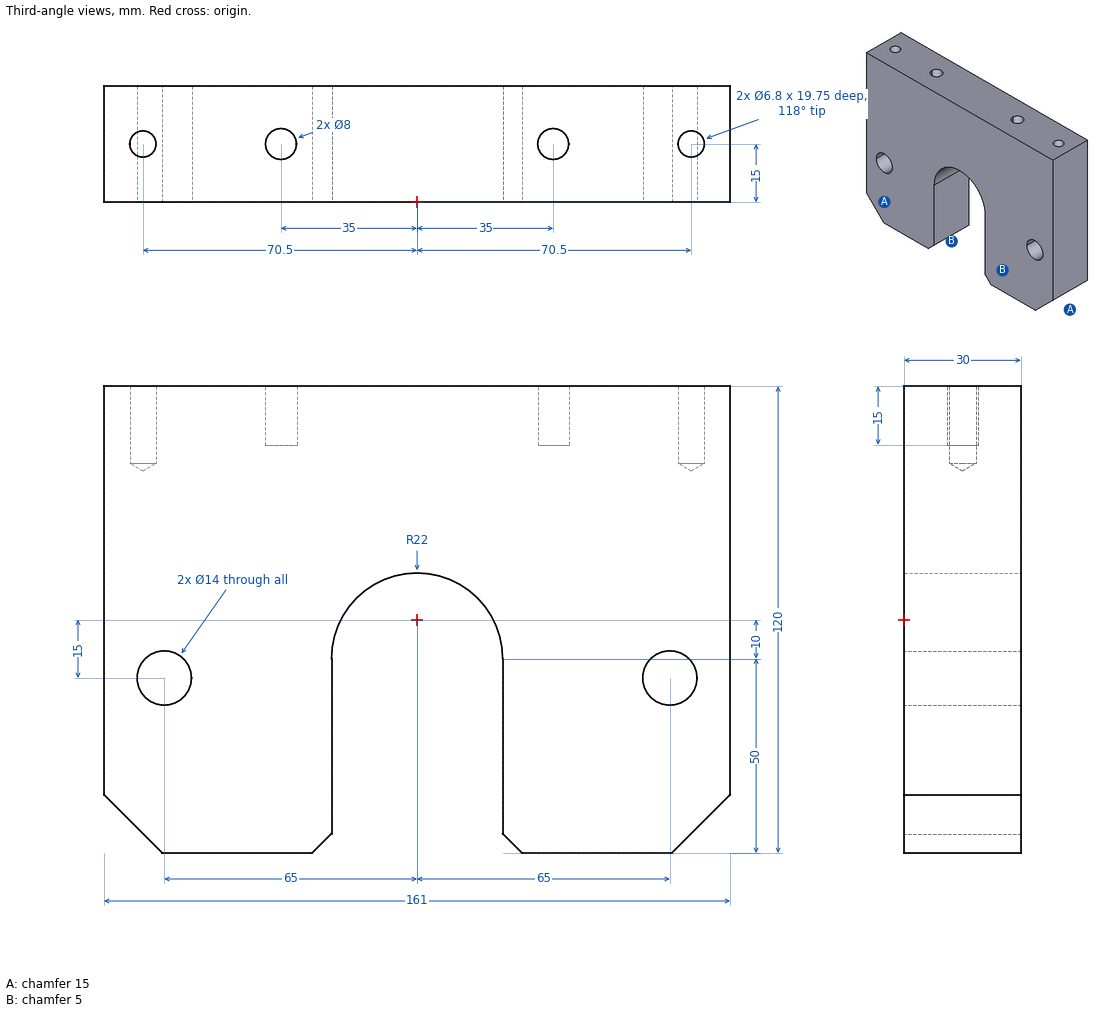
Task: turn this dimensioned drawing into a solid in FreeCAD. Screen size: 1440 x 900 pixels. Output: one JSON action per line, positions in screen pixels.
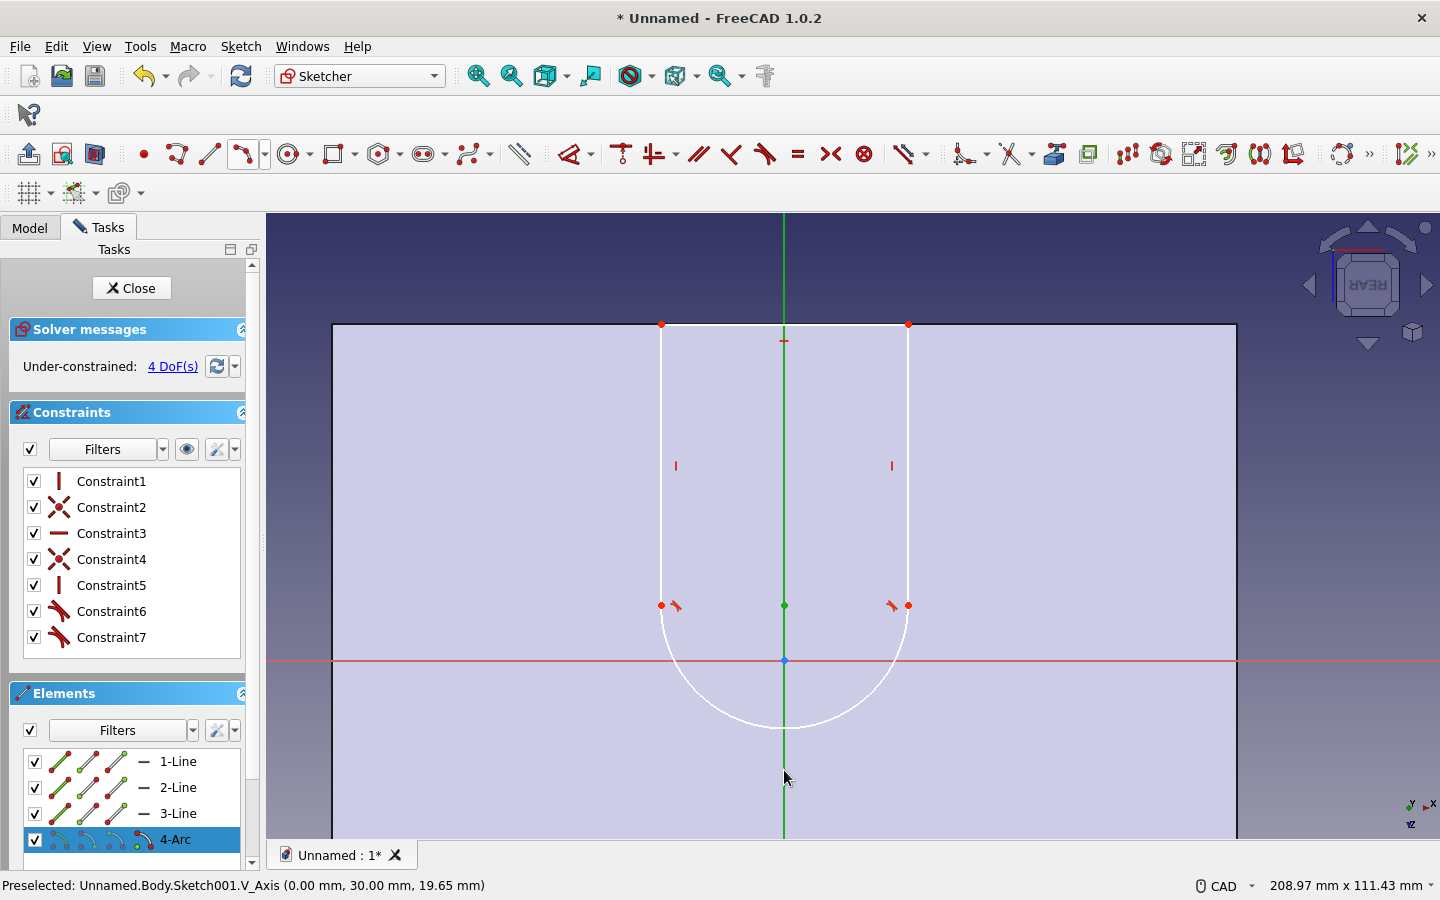
{"action": "key", "text": "c"}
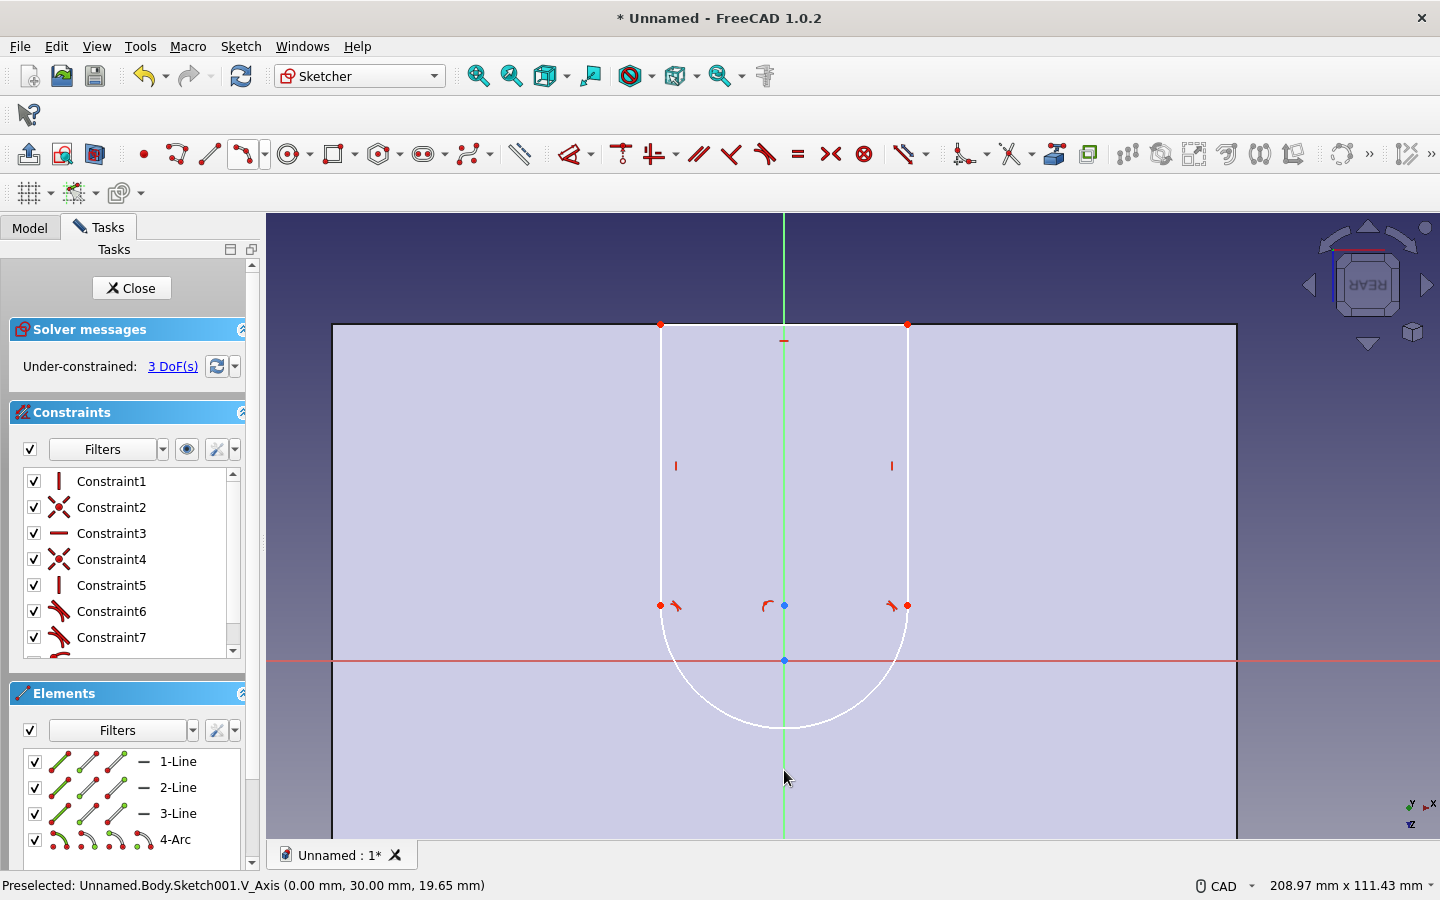
{"action": "key", "text": "d"}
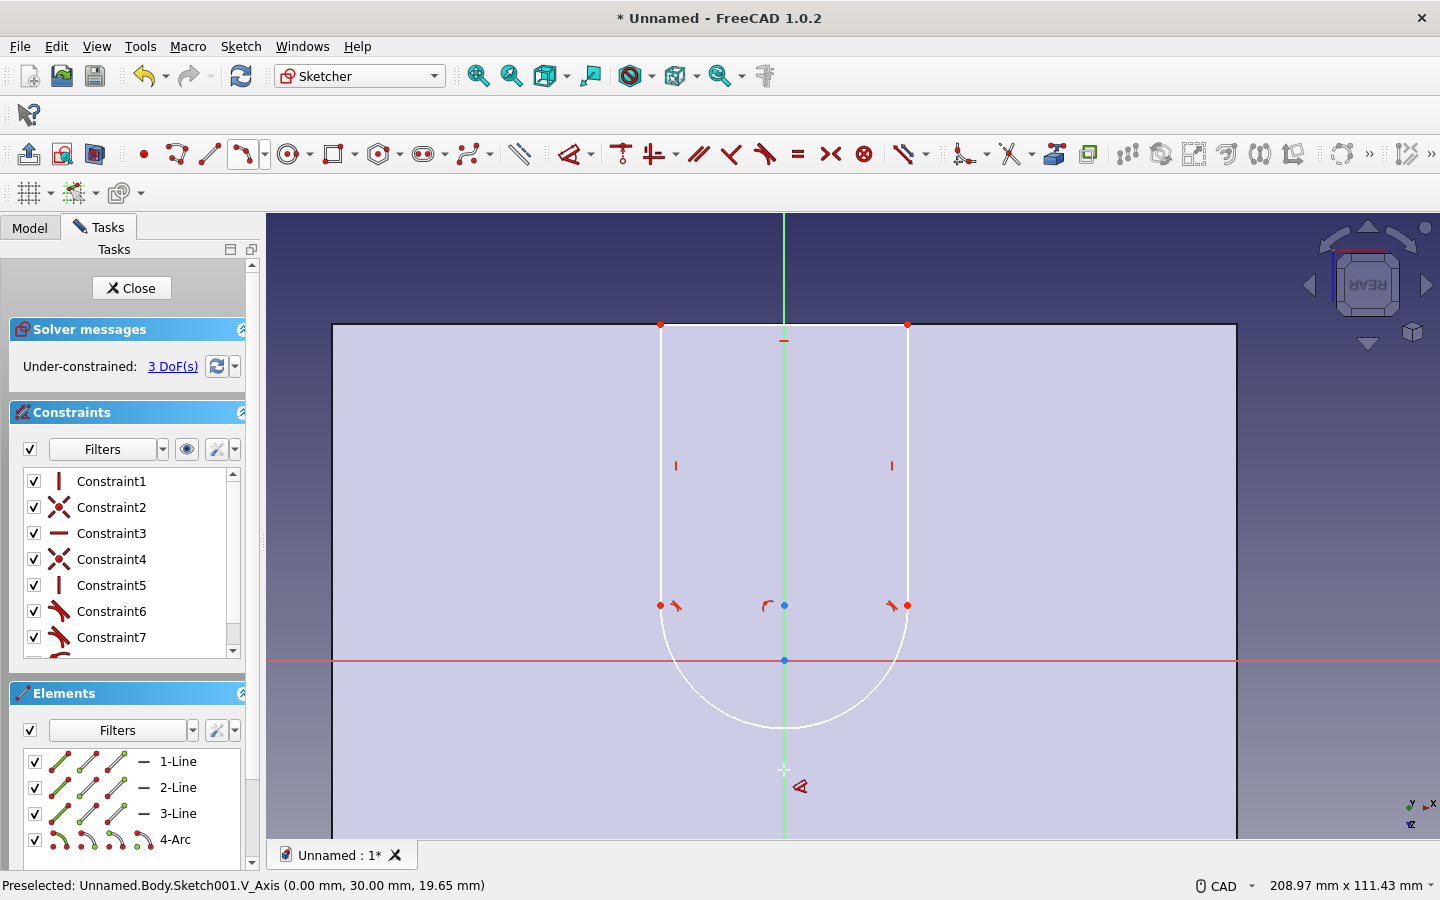
{"action": "left_click", "coordinate": [712, 705]}
{"action": "left_click", "coordinate": [693, 731]}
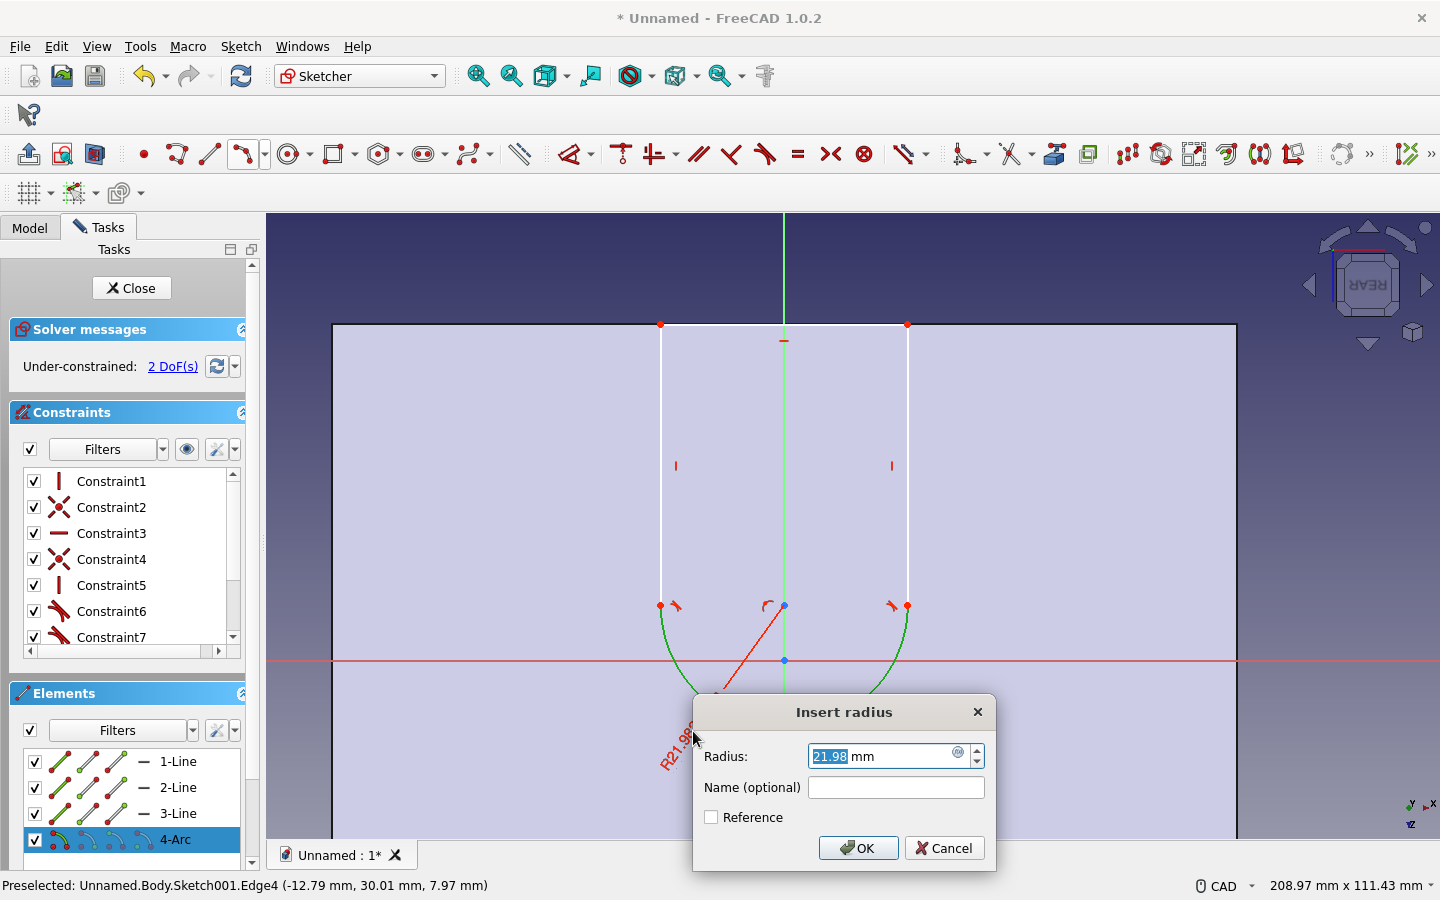
{"action": "type", "text": "22"}
{"action": "key", "text": "Return"}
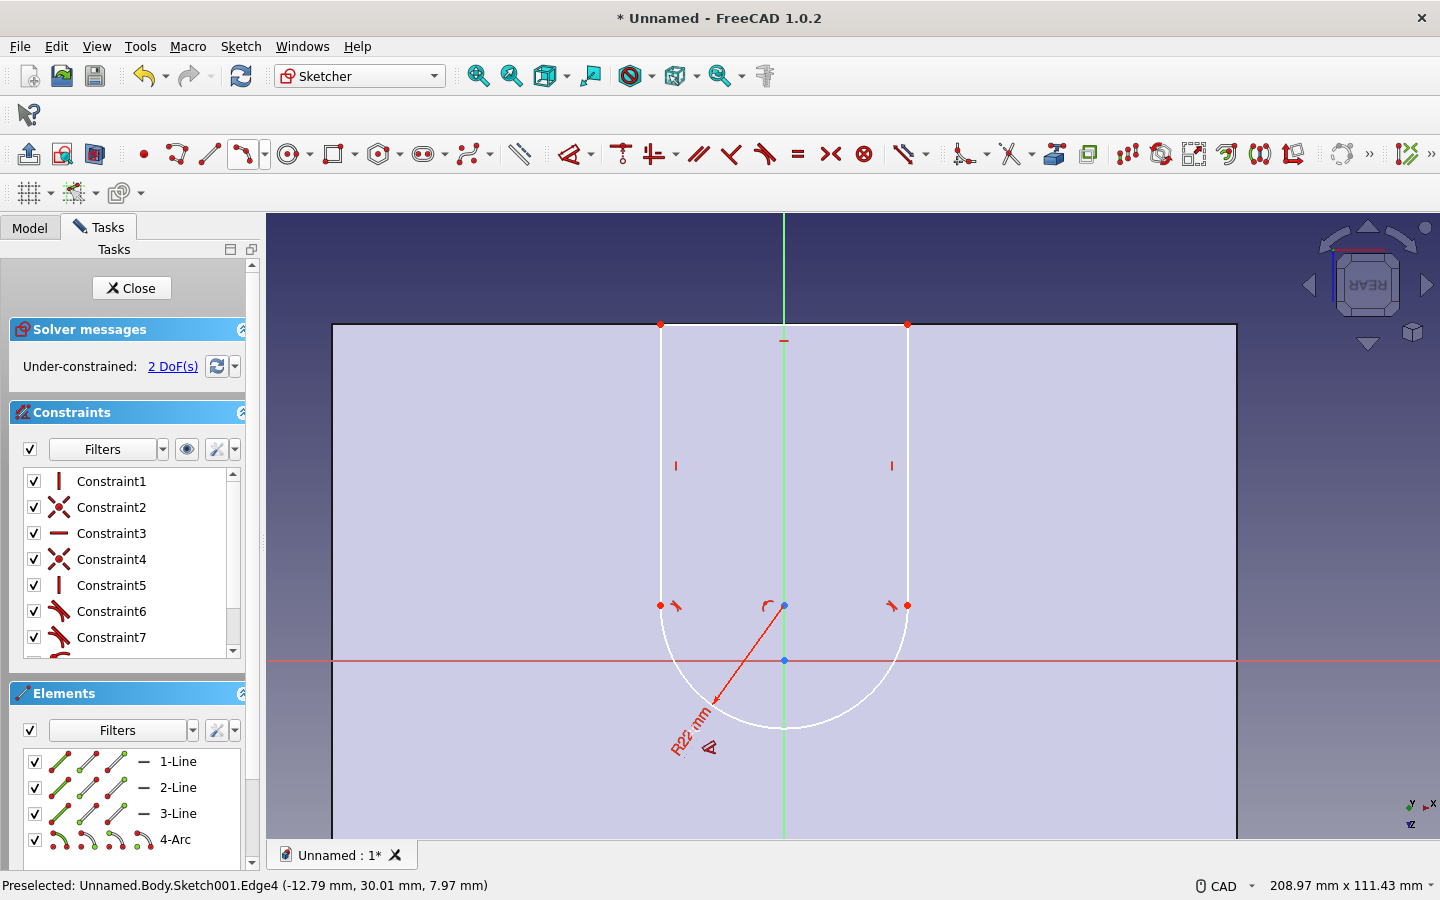
{"action": "left_click", "coordinate": [908, 521]}
{"action": "left_click", "coordinate": [942, 465]}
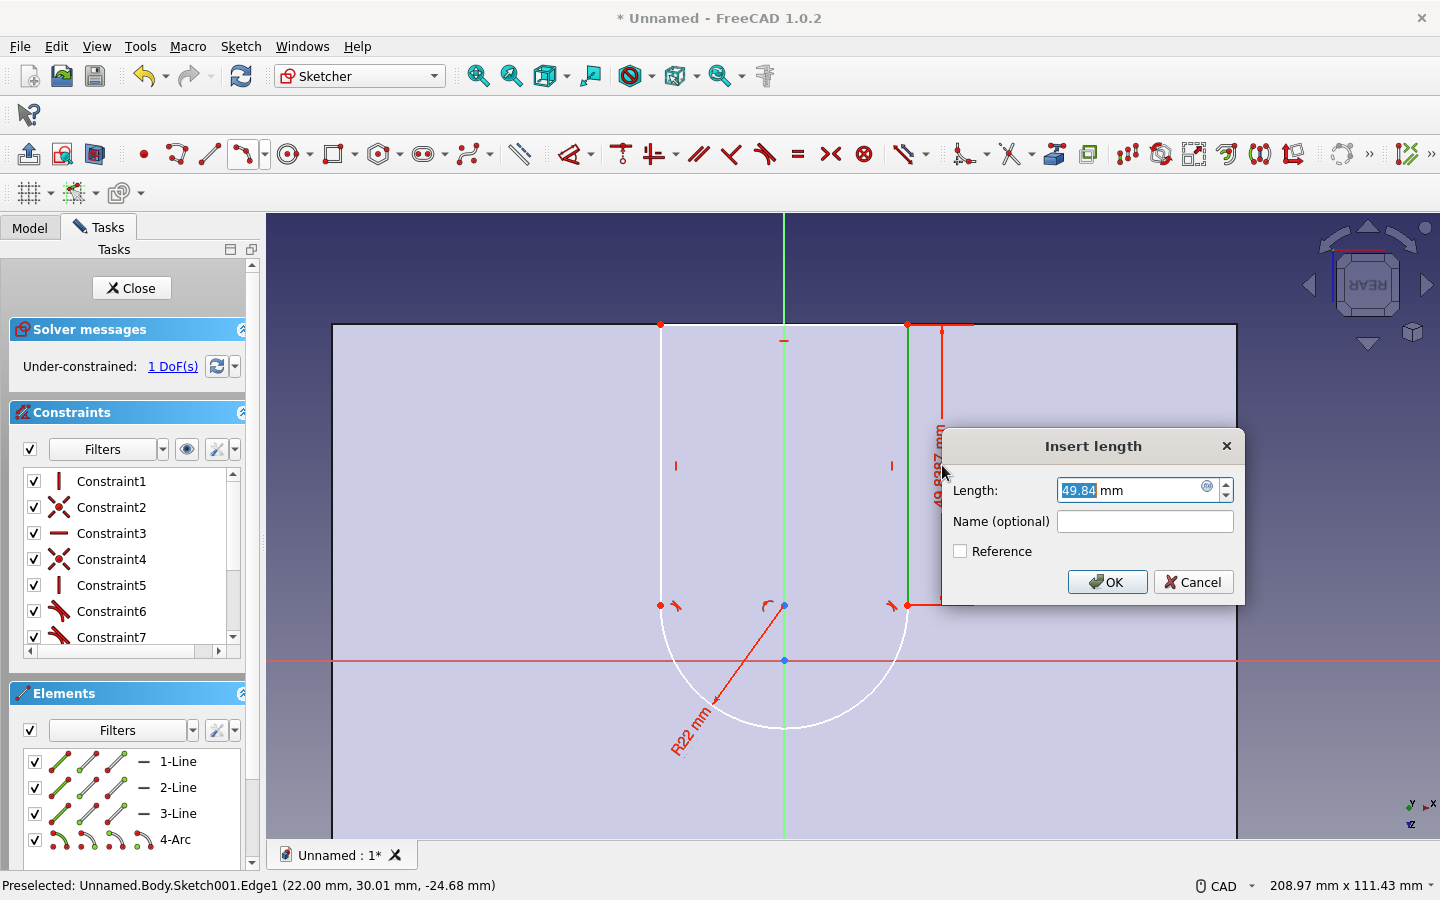
{"action": "type", "text": "50"}
{"action": "key", "text": "Return"}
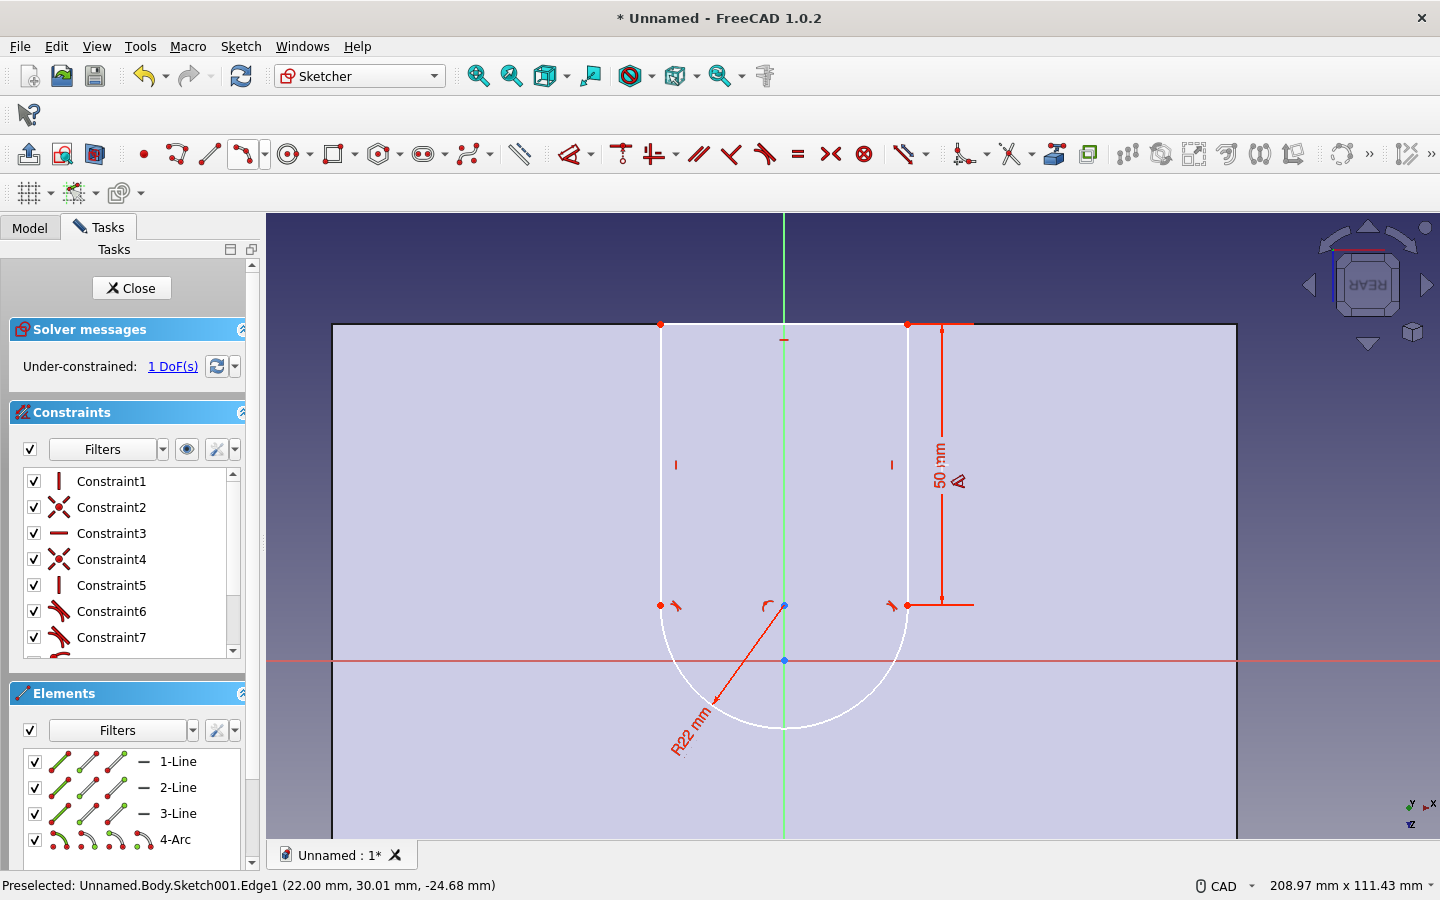
{"action": "left_click", "coordinate": [908, 605]}
{"action": "left_click", "coordinate": [942, 633]}